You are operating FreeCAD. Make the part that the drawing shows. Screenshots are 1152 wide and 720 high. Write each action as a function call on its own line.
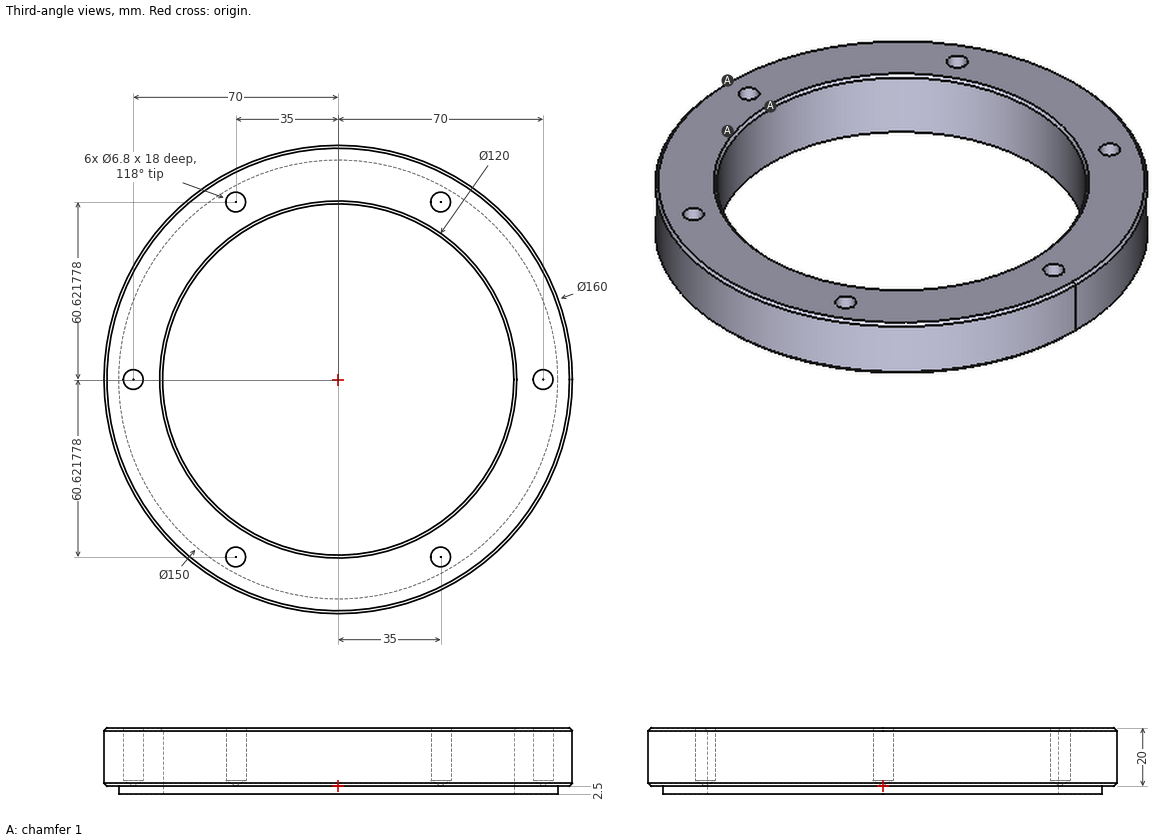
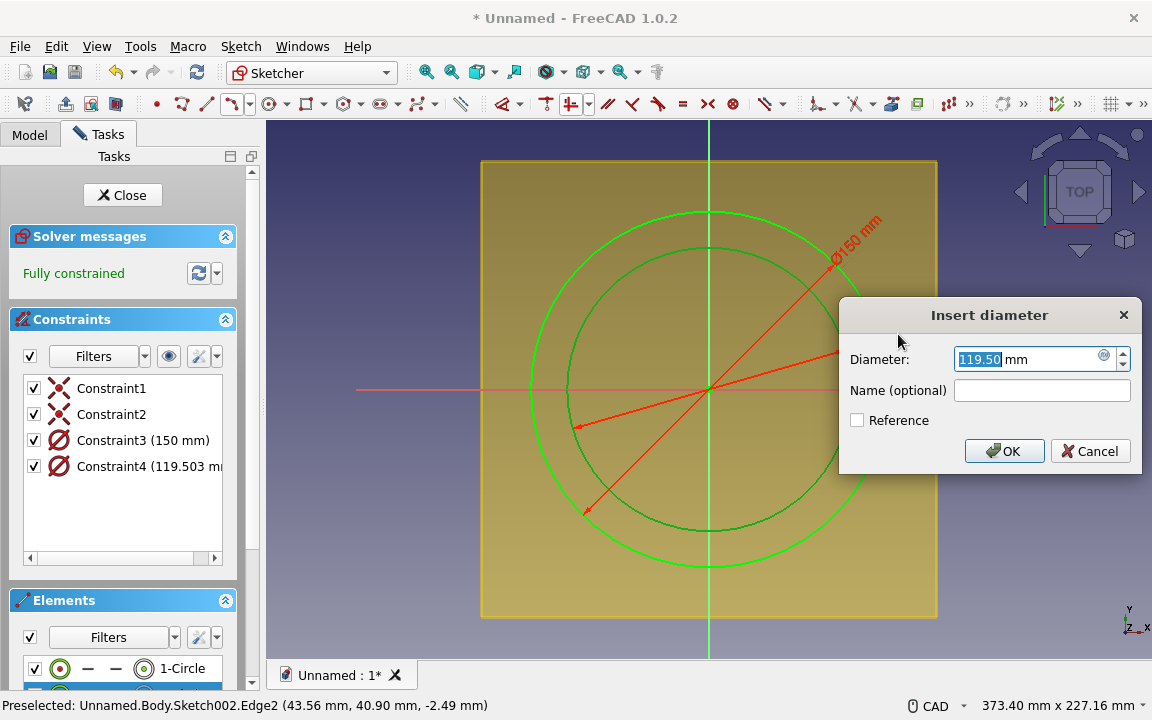
text(120)
key(Return)
key(Escape)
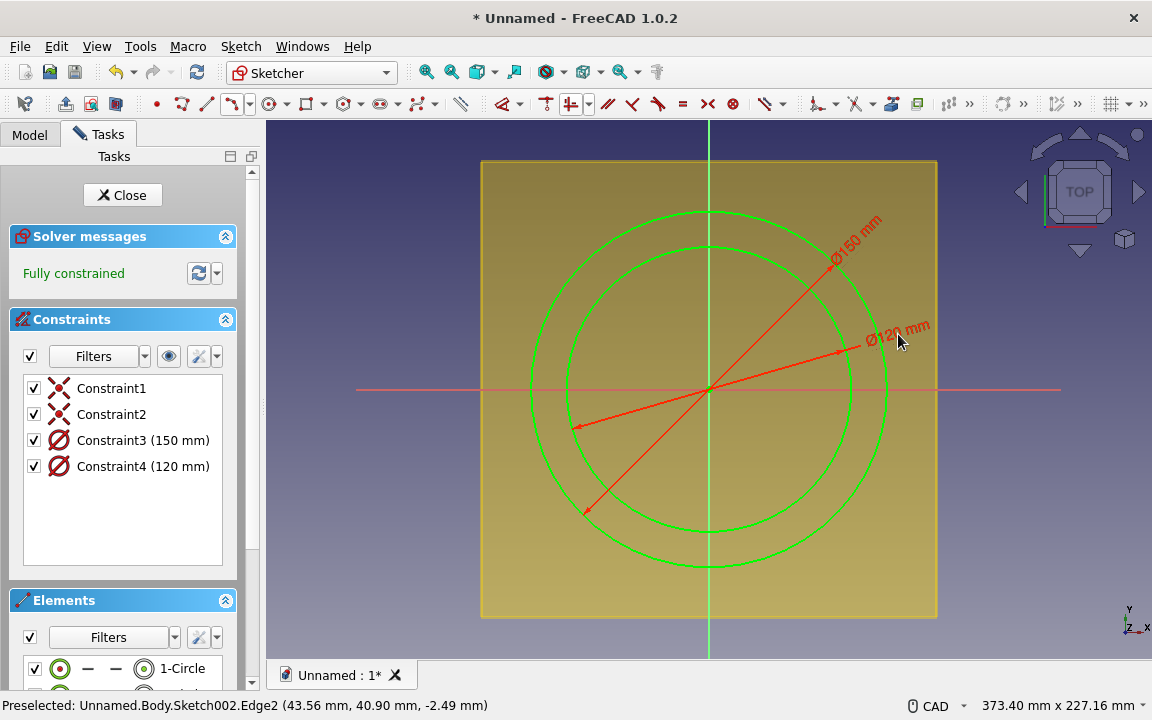
click(123, 195)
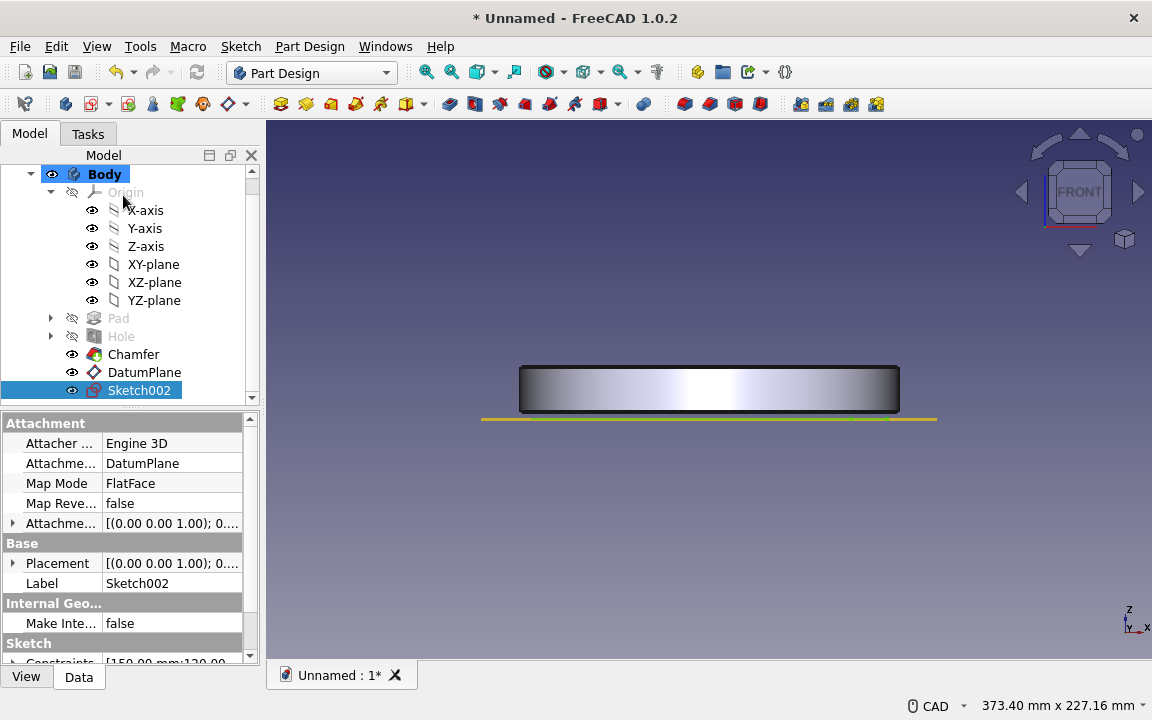
click(281, 104)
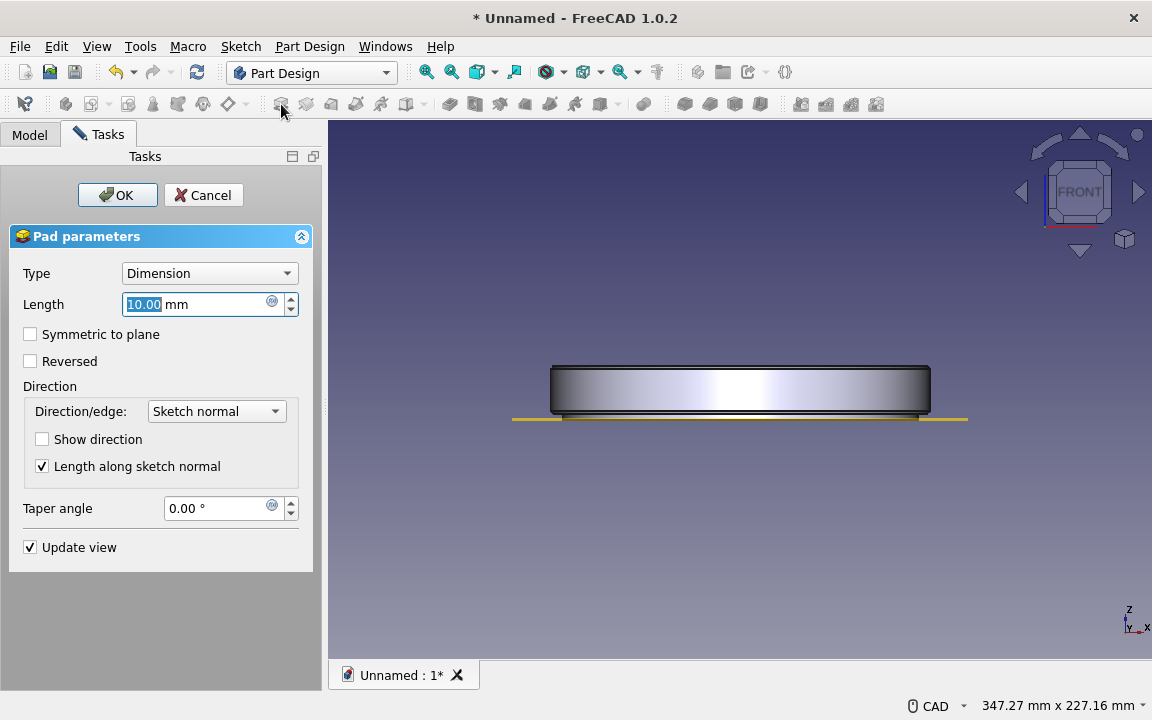
text(2.5)
key(Tab)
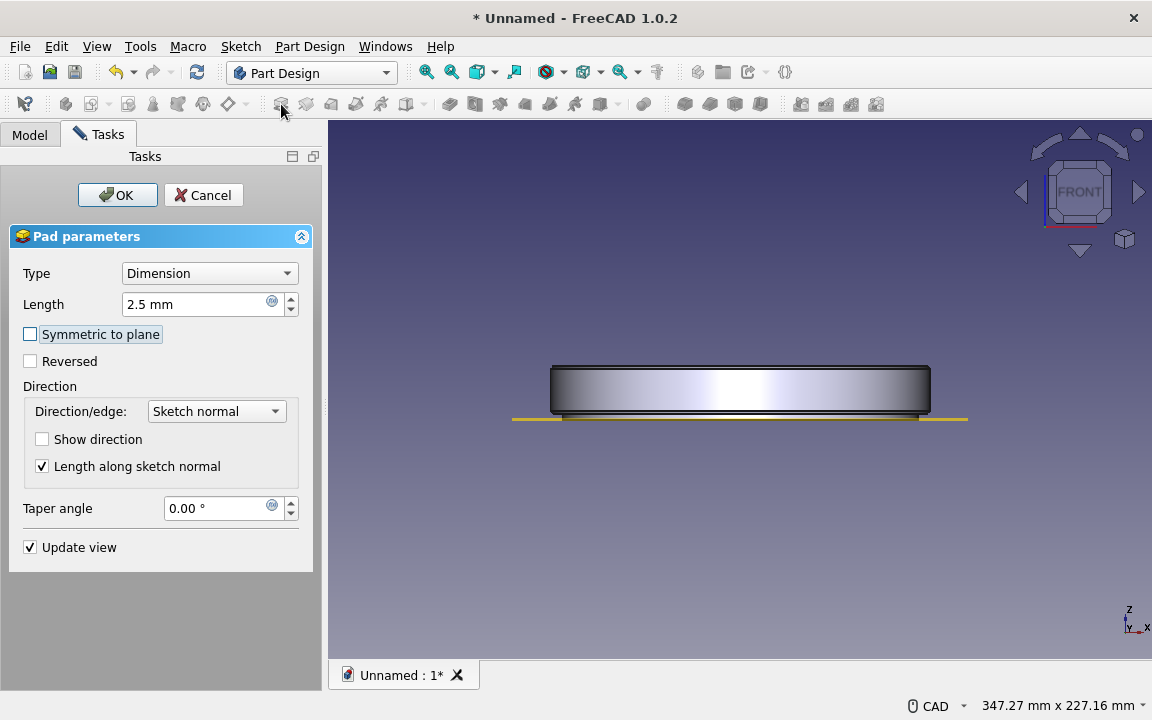
click(118, 195)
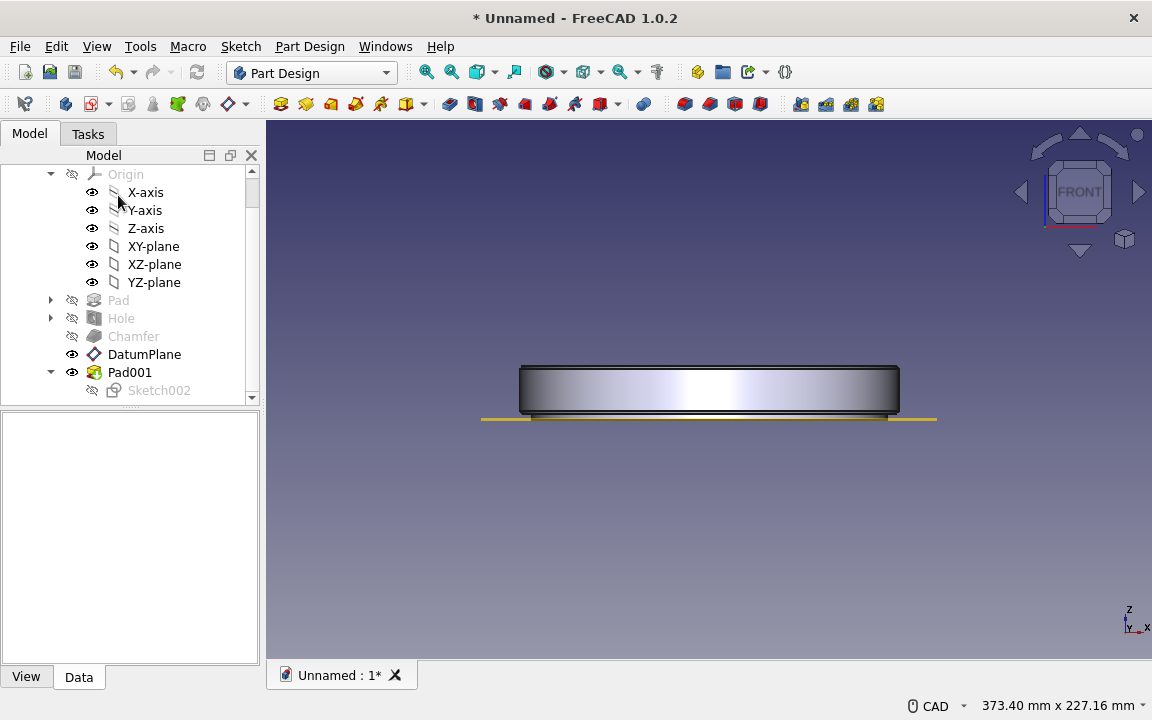
click(117, 354)
key(space)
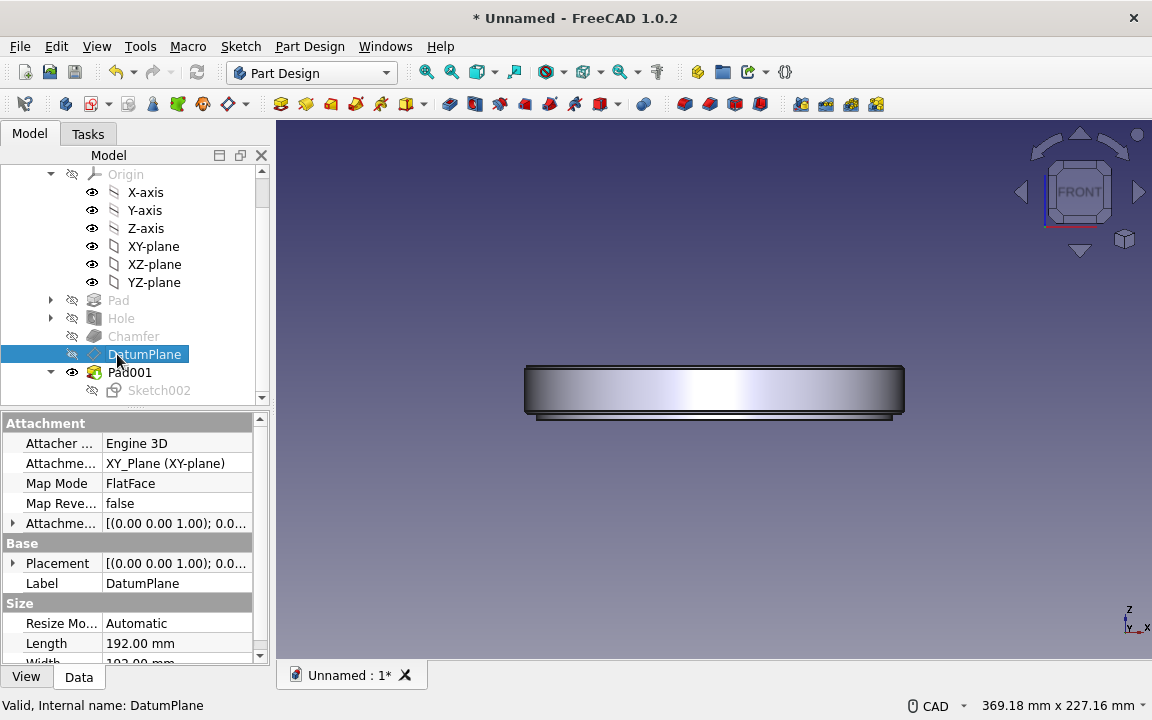
key(0)